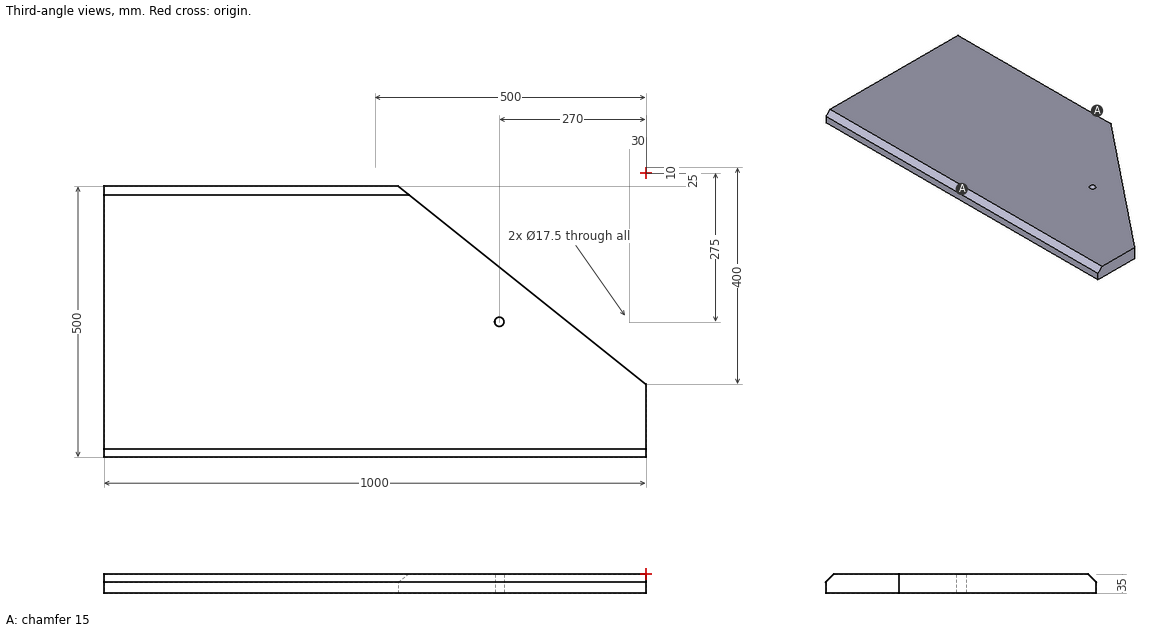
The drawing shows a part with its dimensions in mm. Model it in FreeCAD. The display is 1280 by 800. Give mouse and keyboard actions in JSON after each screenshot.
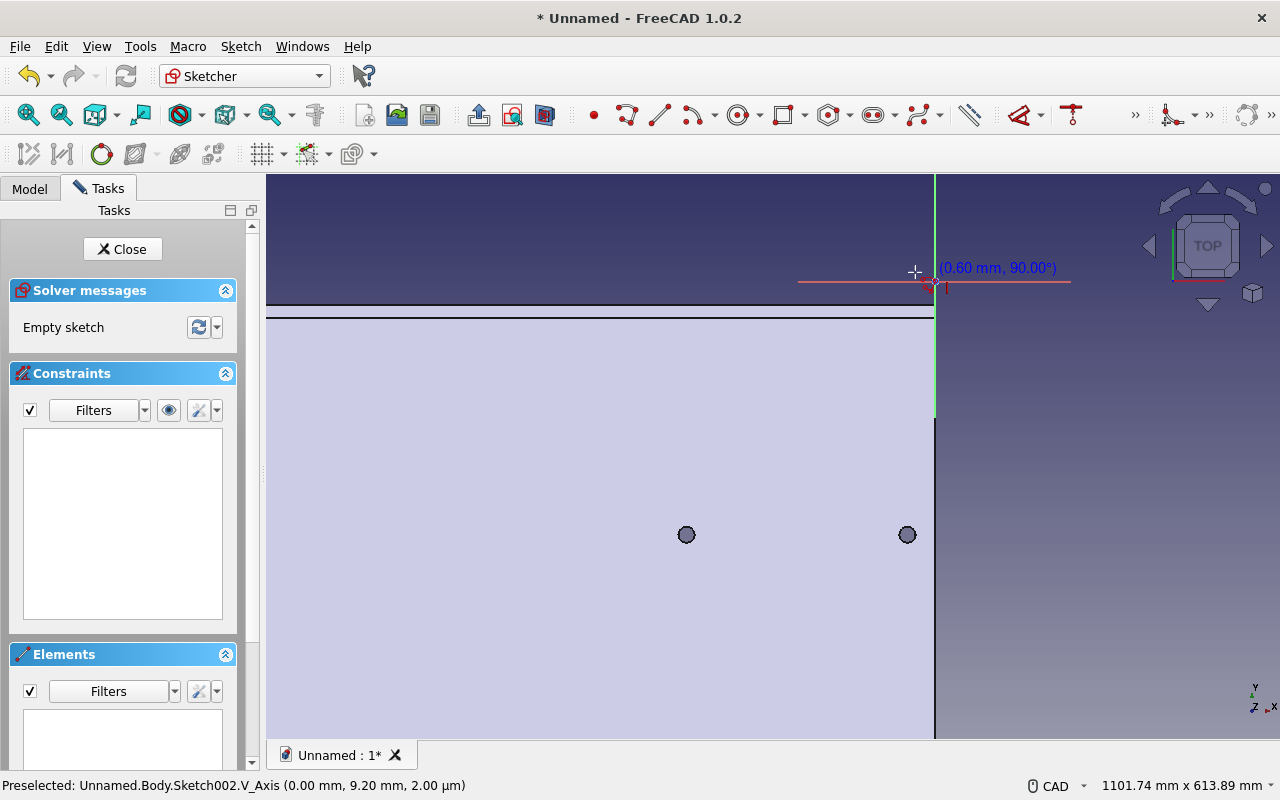
{"action": "scroll", "coordinate": [475, 272], "scroll_direction": "up", "scroll_amount": 3}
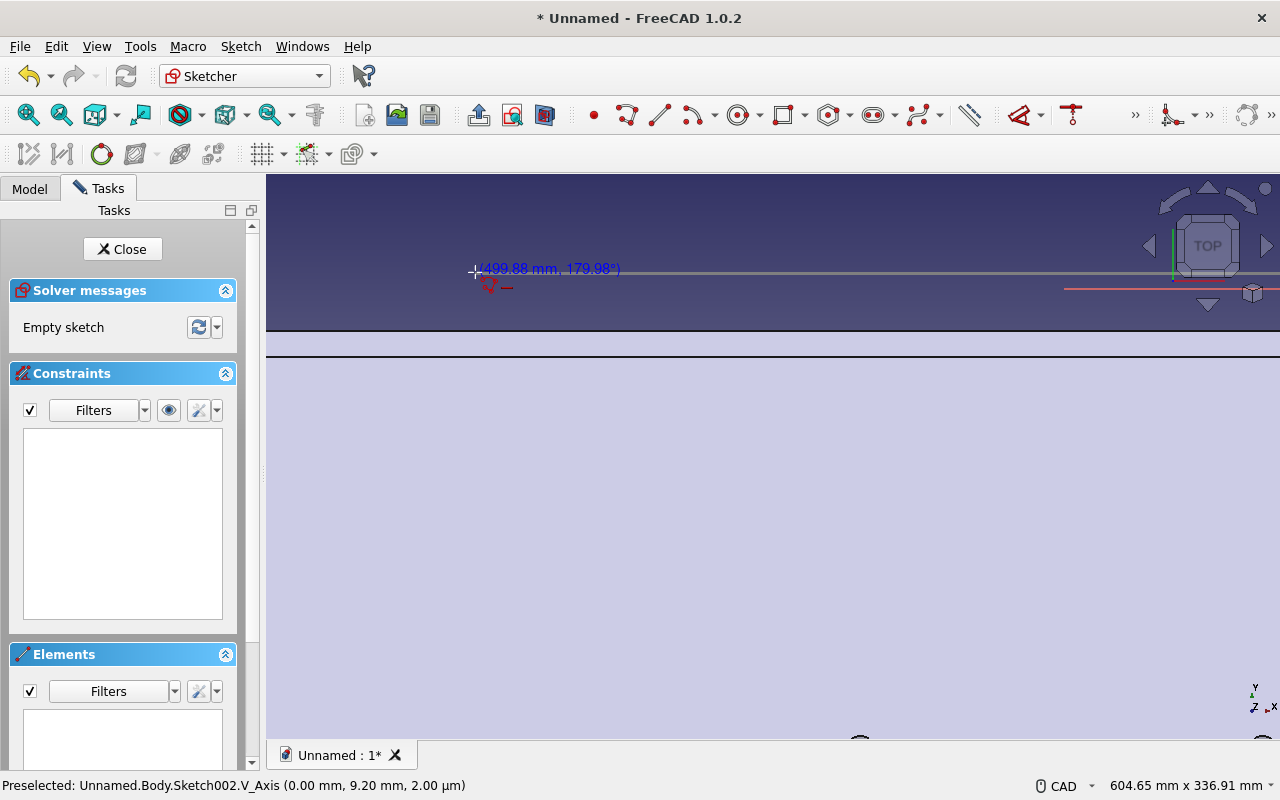
{"action": "left_click", "coordinate": [475, 273]}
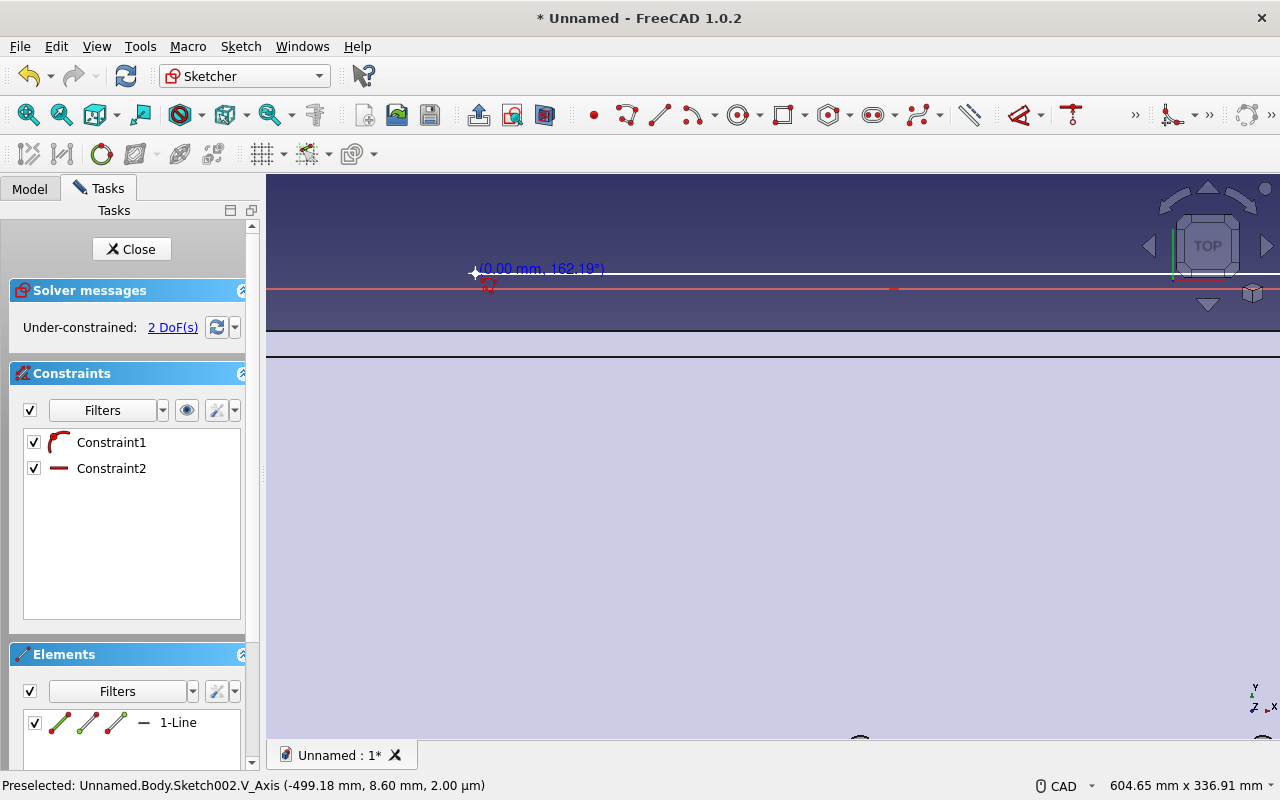
{"action": "scroll", "coordinate": [474, 272], "scroll_direction": "down", "scroll_amount": 3}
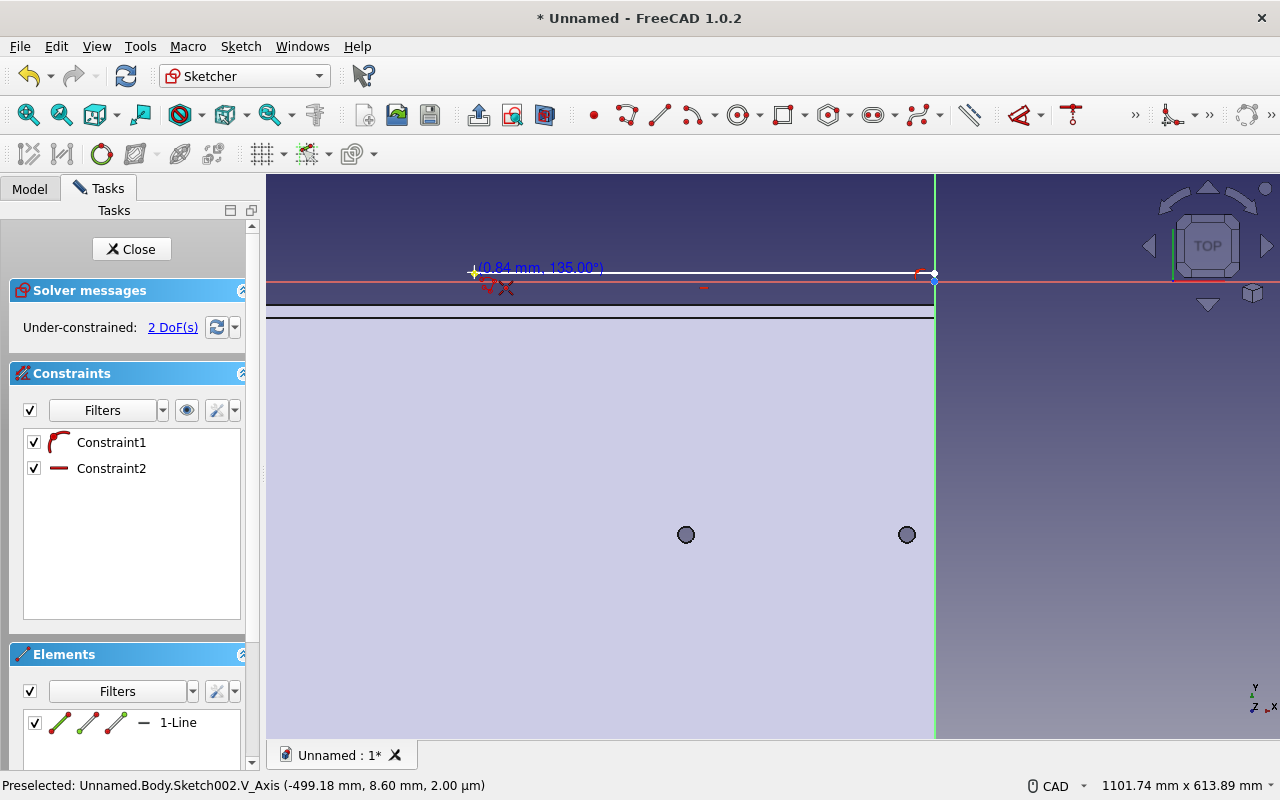
{"action": "left_click", "coordinate": [926, 641]}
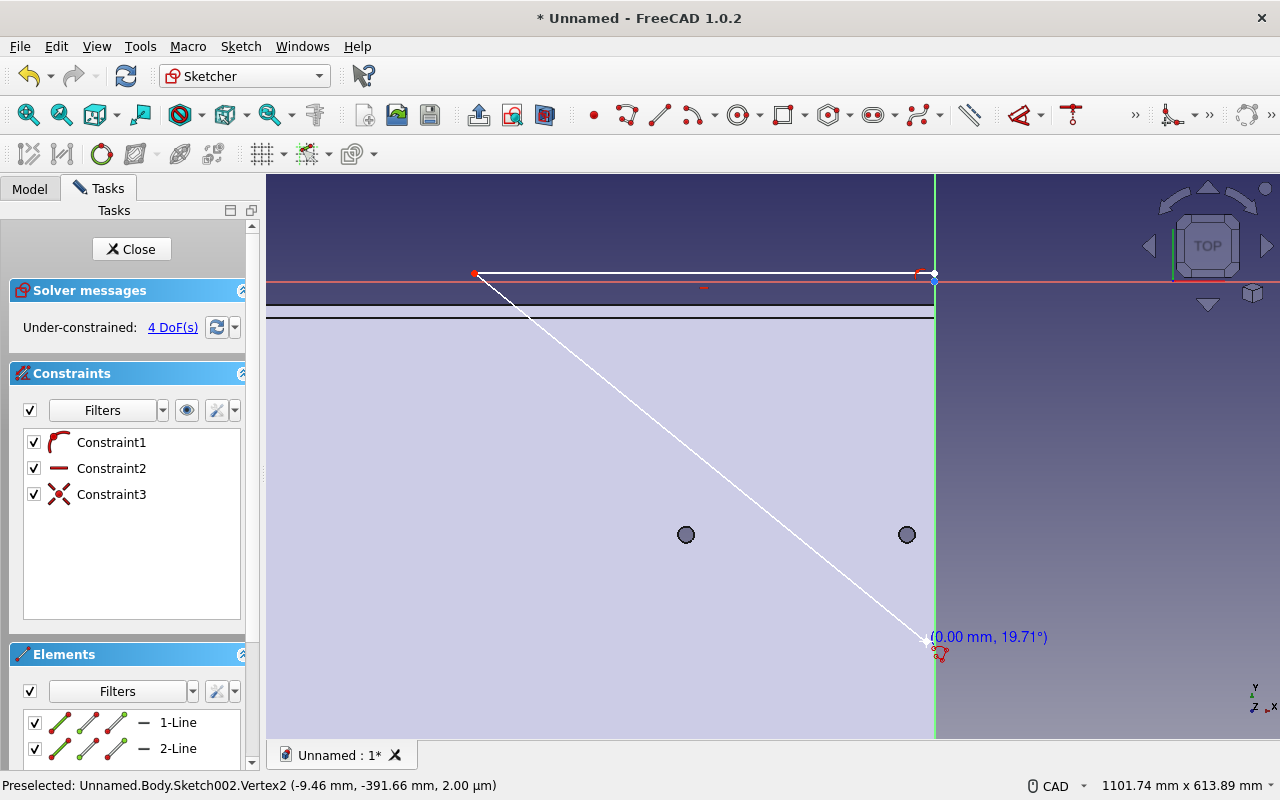
{"action": "scroll", "coordinate": [935, 272], "scroll_direction": "up", "scroll_amount": 3}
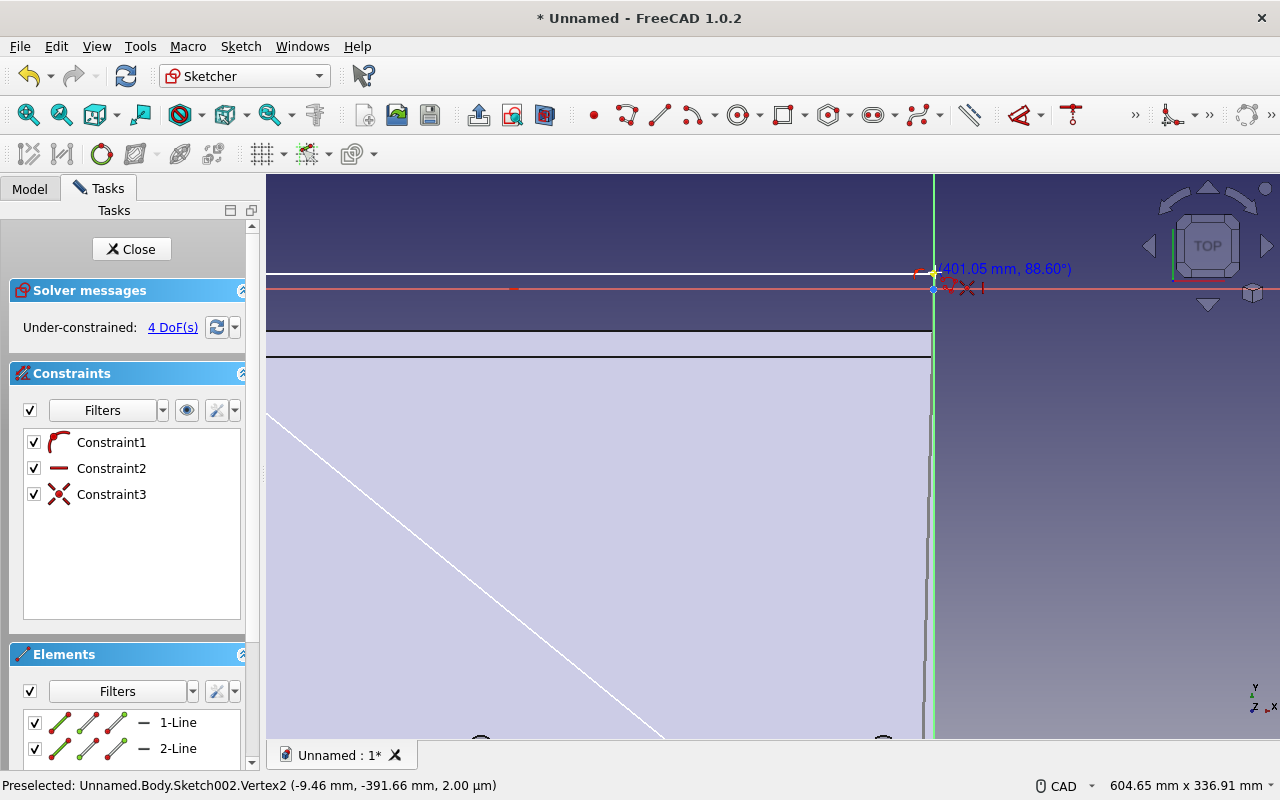
{"action": "left_click", "coordinate": [934, 274]}
{"action": "key", "text": "Escape"}
{"action": "key", "text": "Escape"}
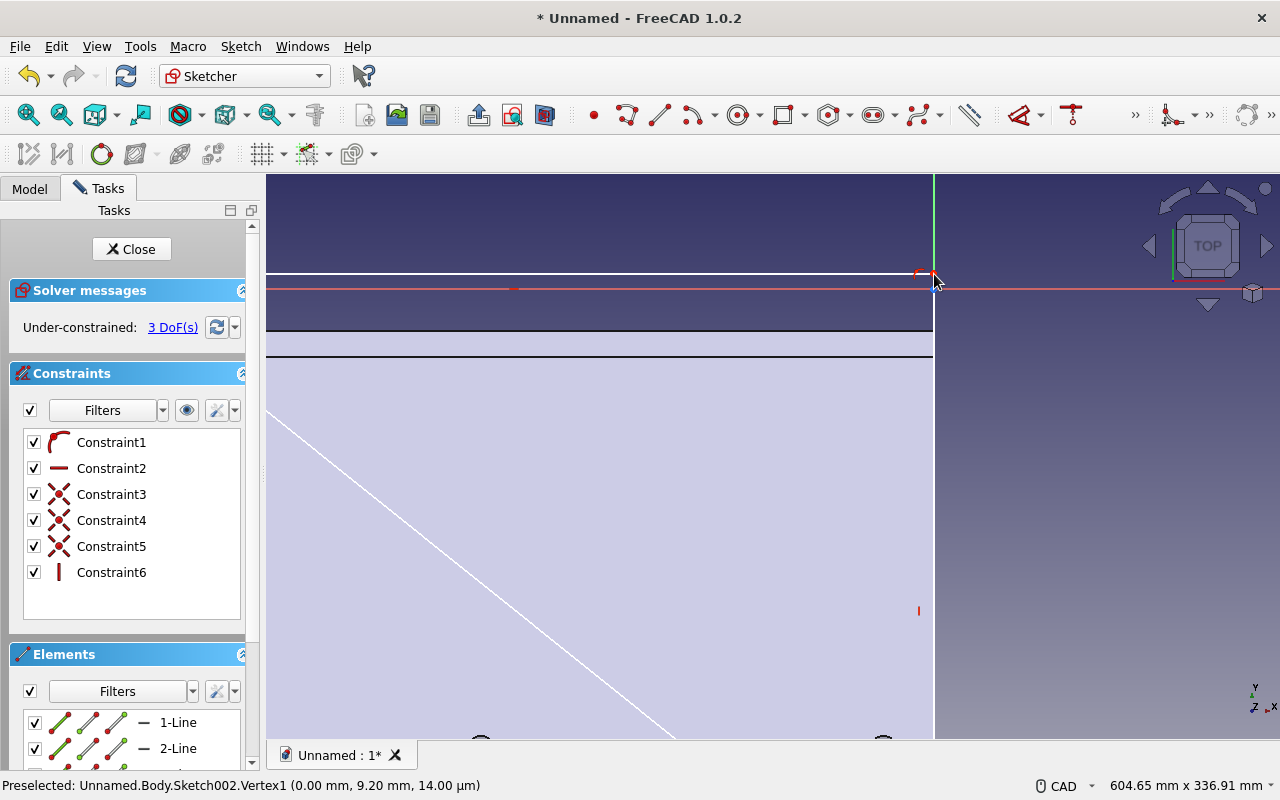
{"action": "left_click", "coordinate": [1018, 116]}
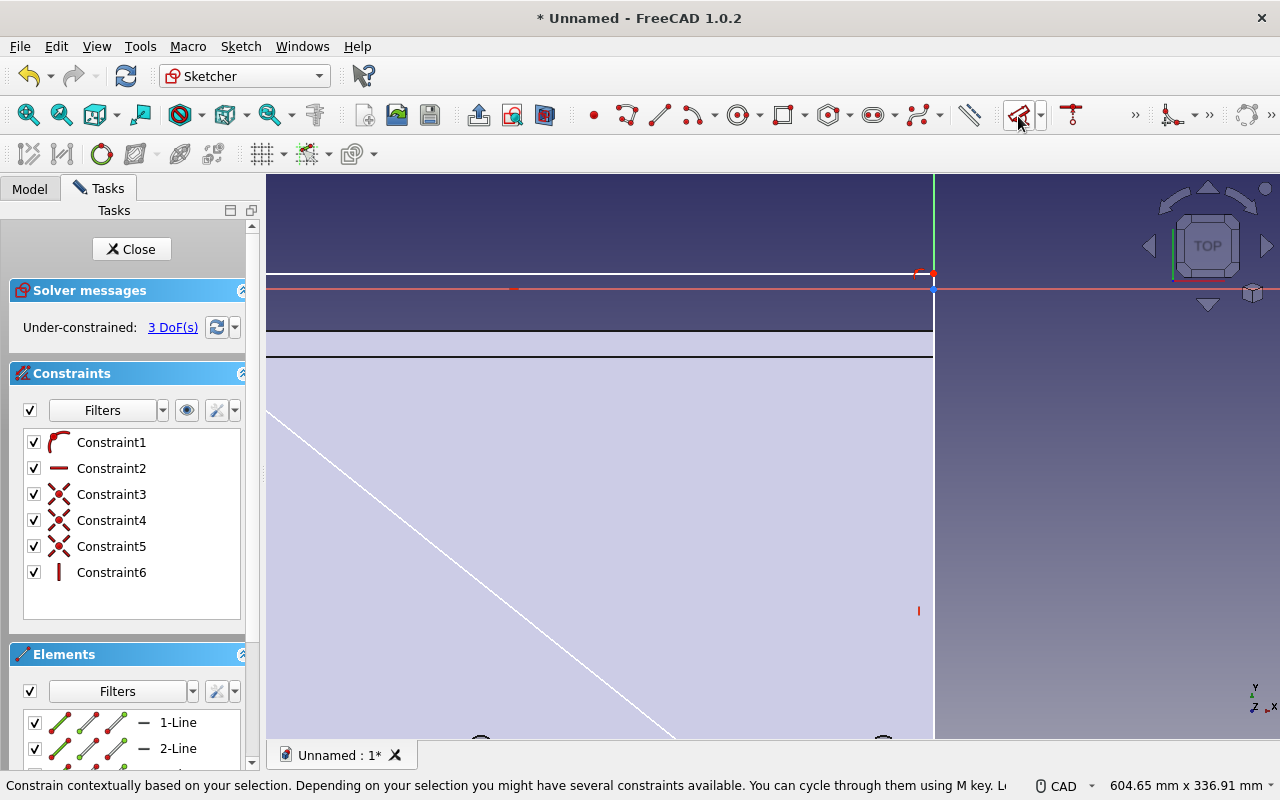
{"action": "left_click", "coordinate": [682, 274]}
{"action": "left_click", "coordinate": [614, 240]}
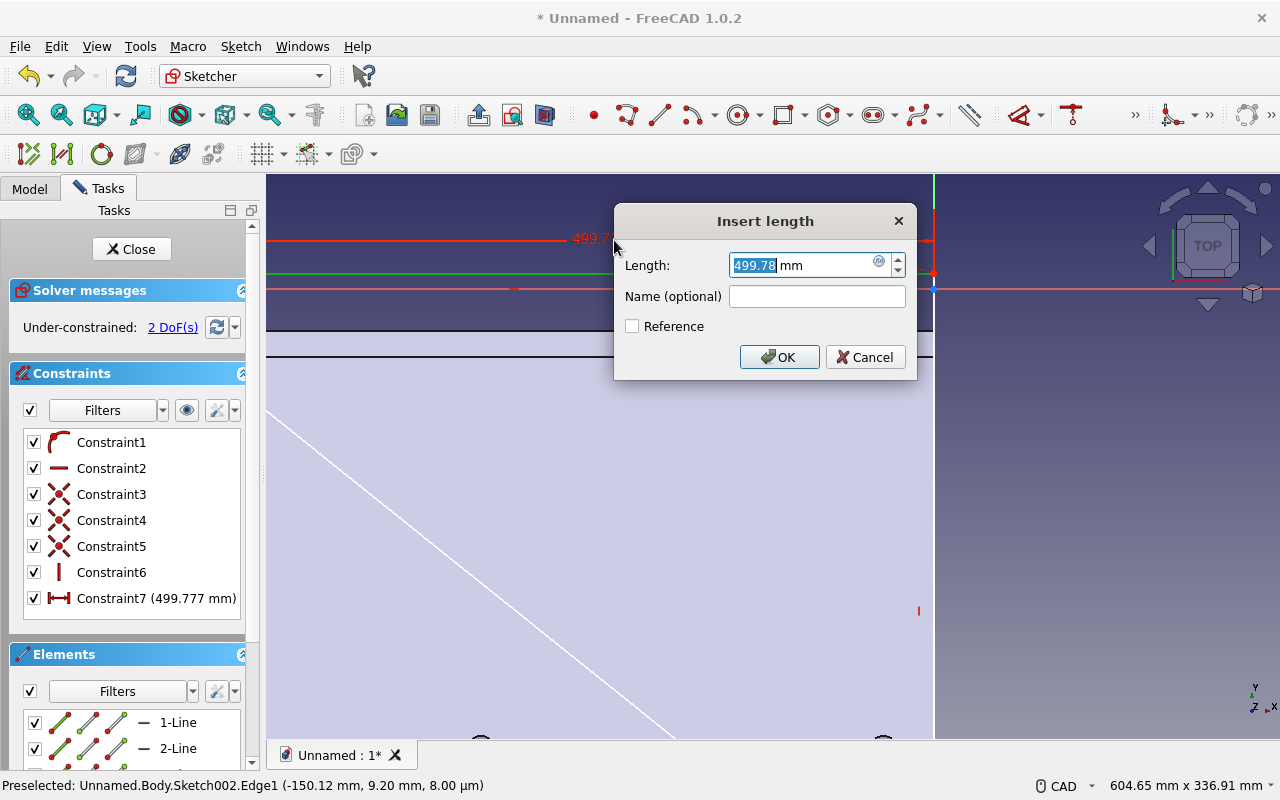
{"action": "type", "text": "500"}
{"action": "key", "text": "Return"}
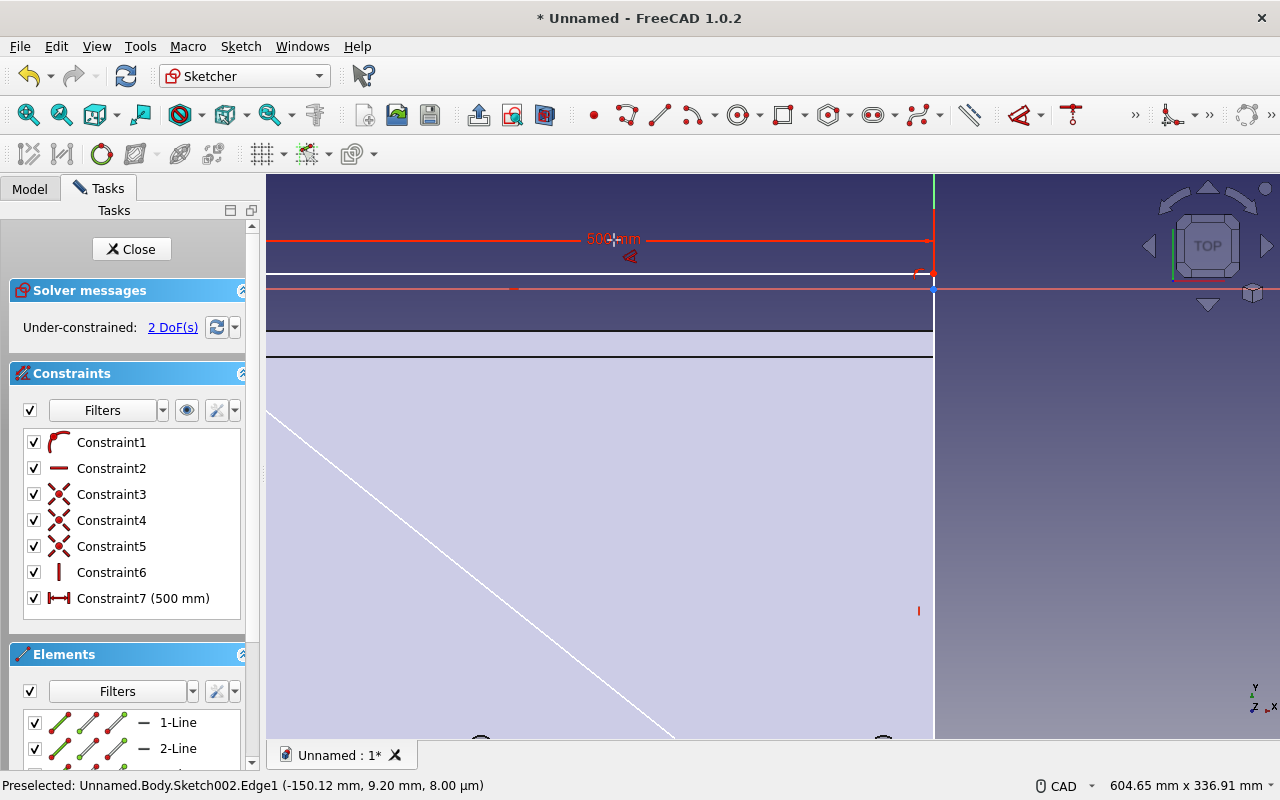
{"action": "left_click", "coordinate": [934, 476]}
{"action": "left_click", "coordinate": [968, 493]}